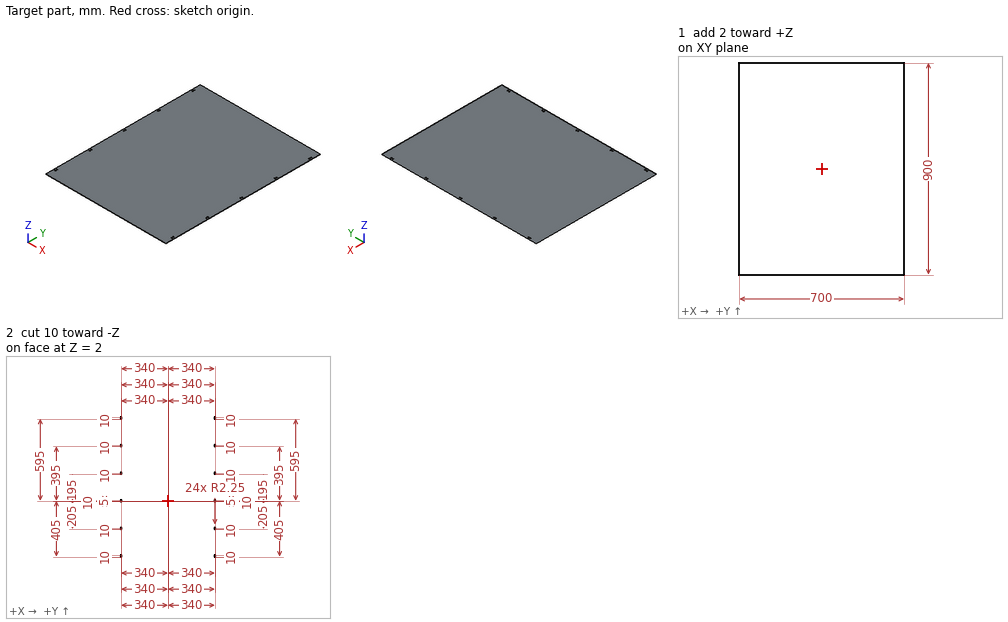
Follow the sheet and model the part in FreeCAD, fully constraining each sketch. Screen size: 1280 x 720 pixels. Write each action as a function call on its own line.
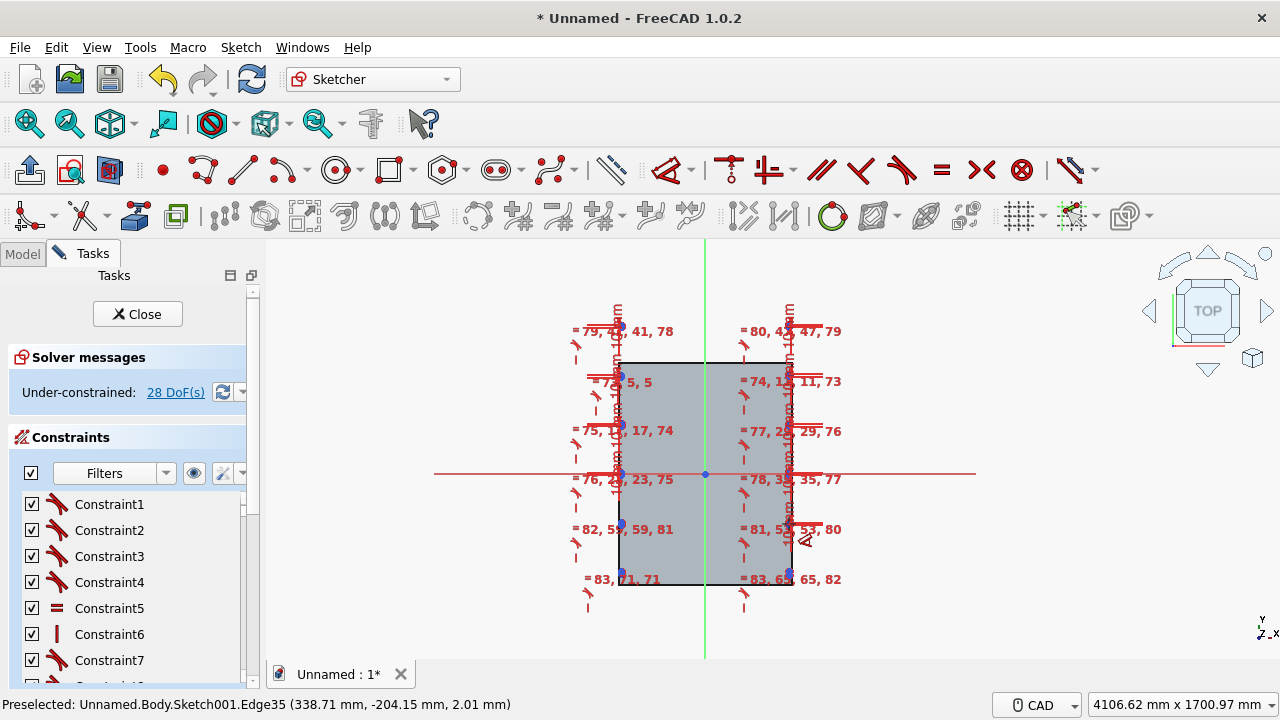
scroll(621, 524, up, 14)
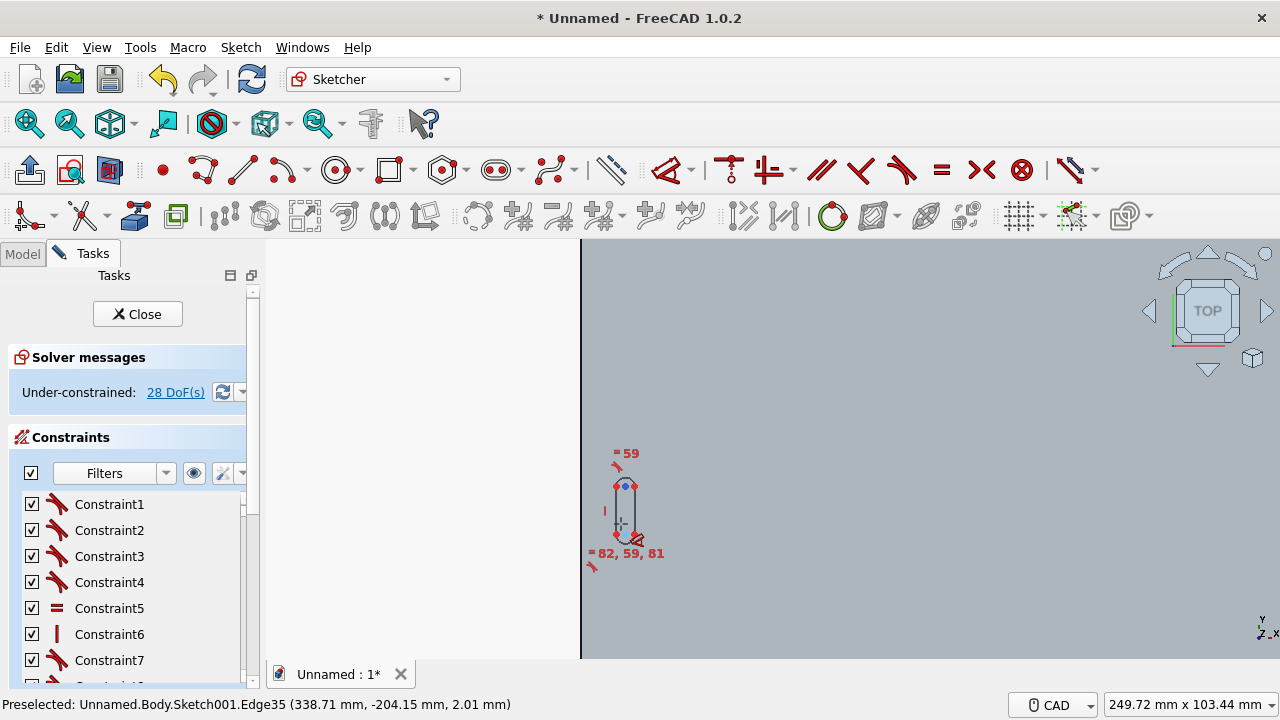
click(616, 520)
click(582, 511)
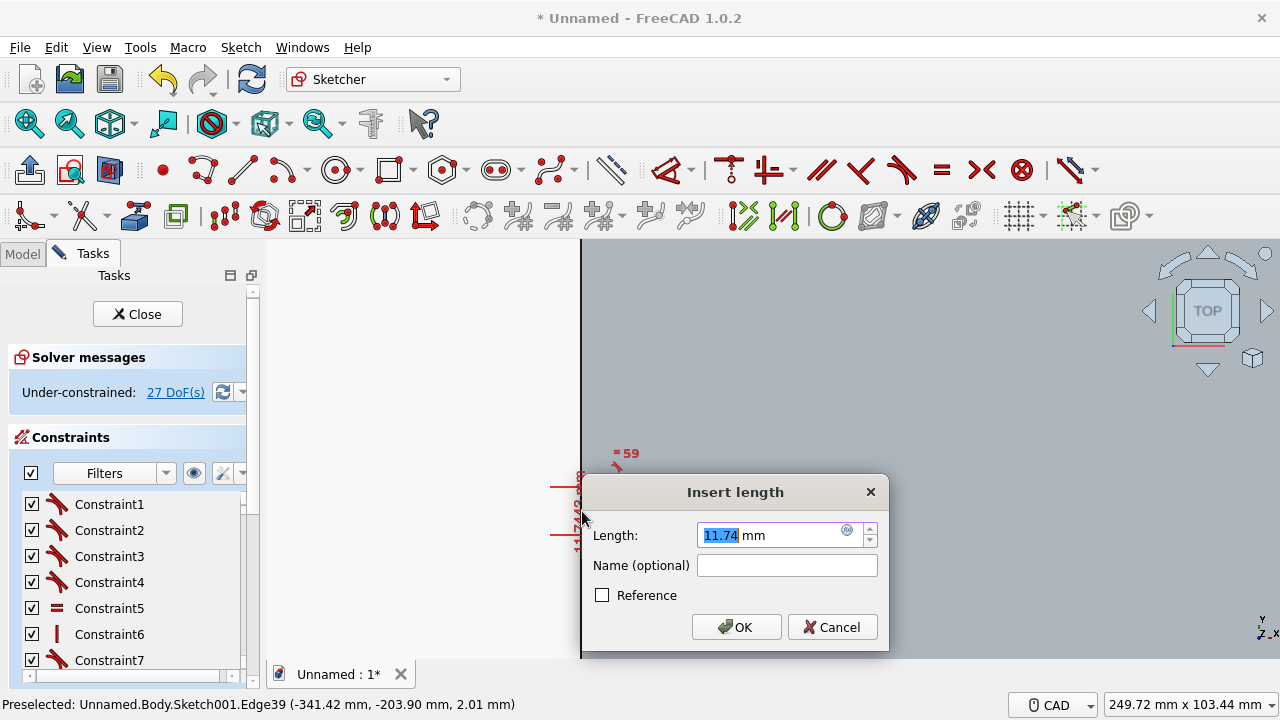
text(10)
key(Return)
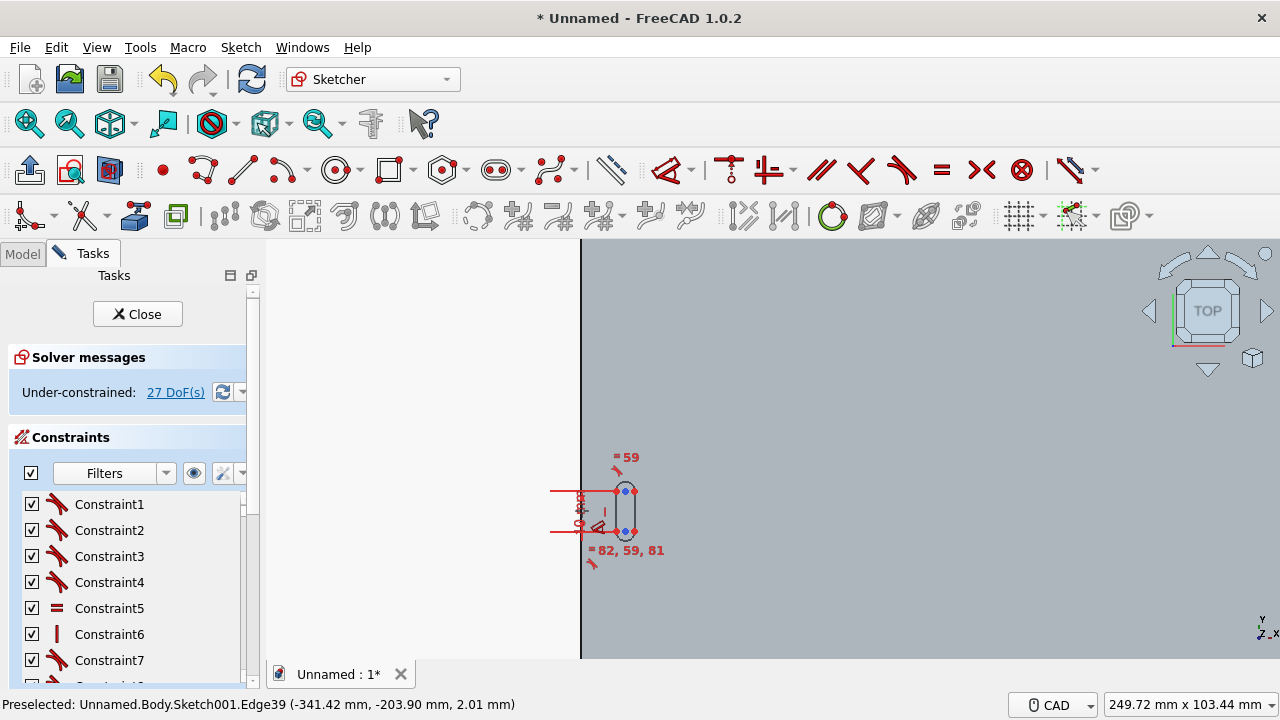
scroll(620, 524, down, 14)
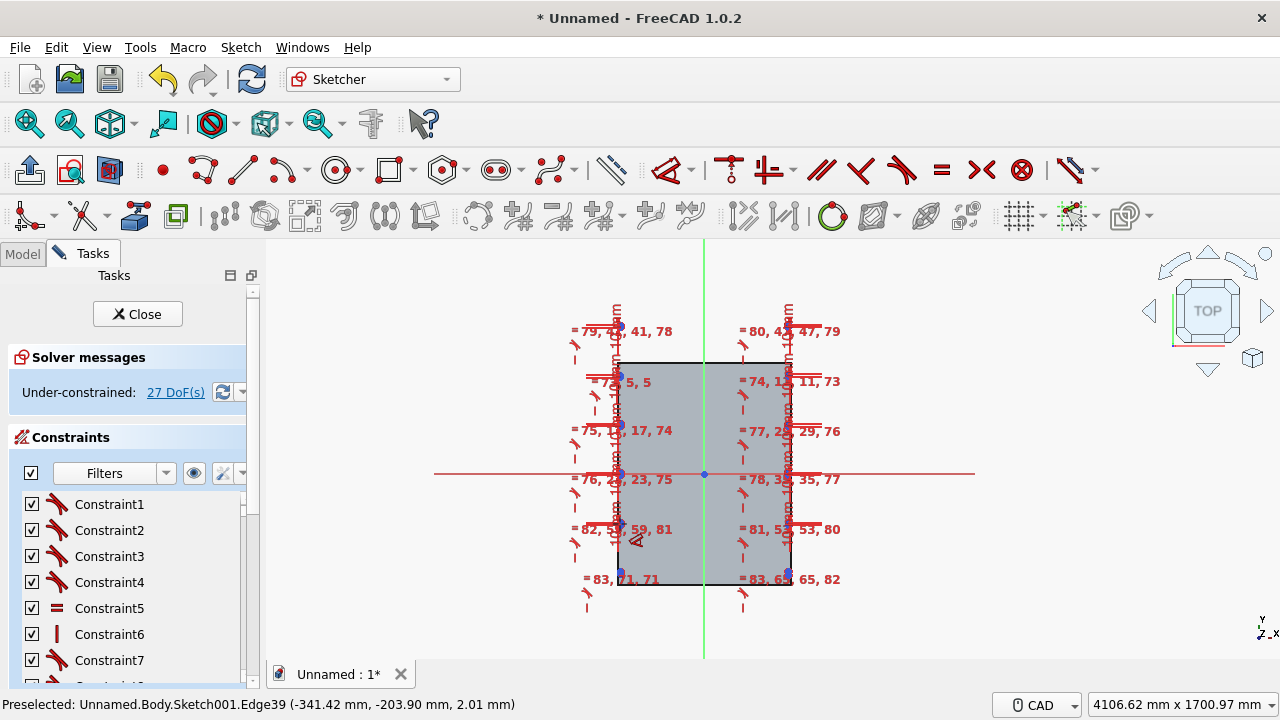
scroll(788, 574, up, 14)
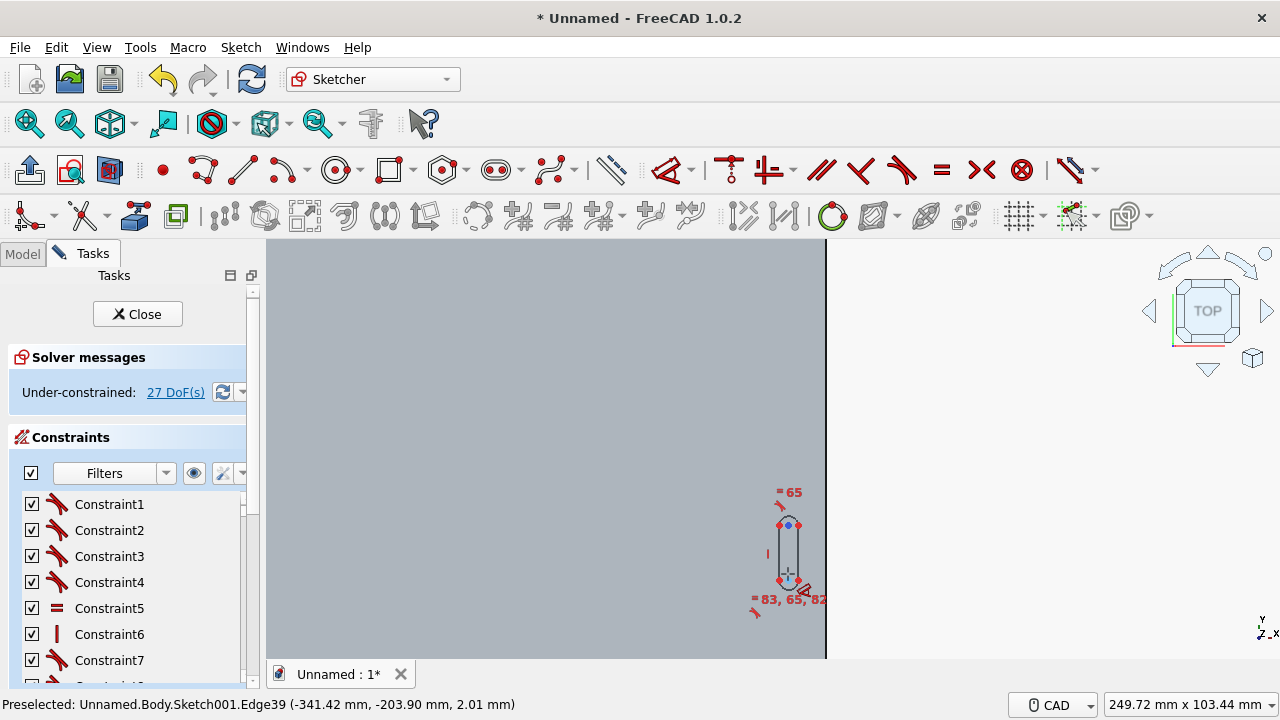
click(779, 564)
click(813, 553)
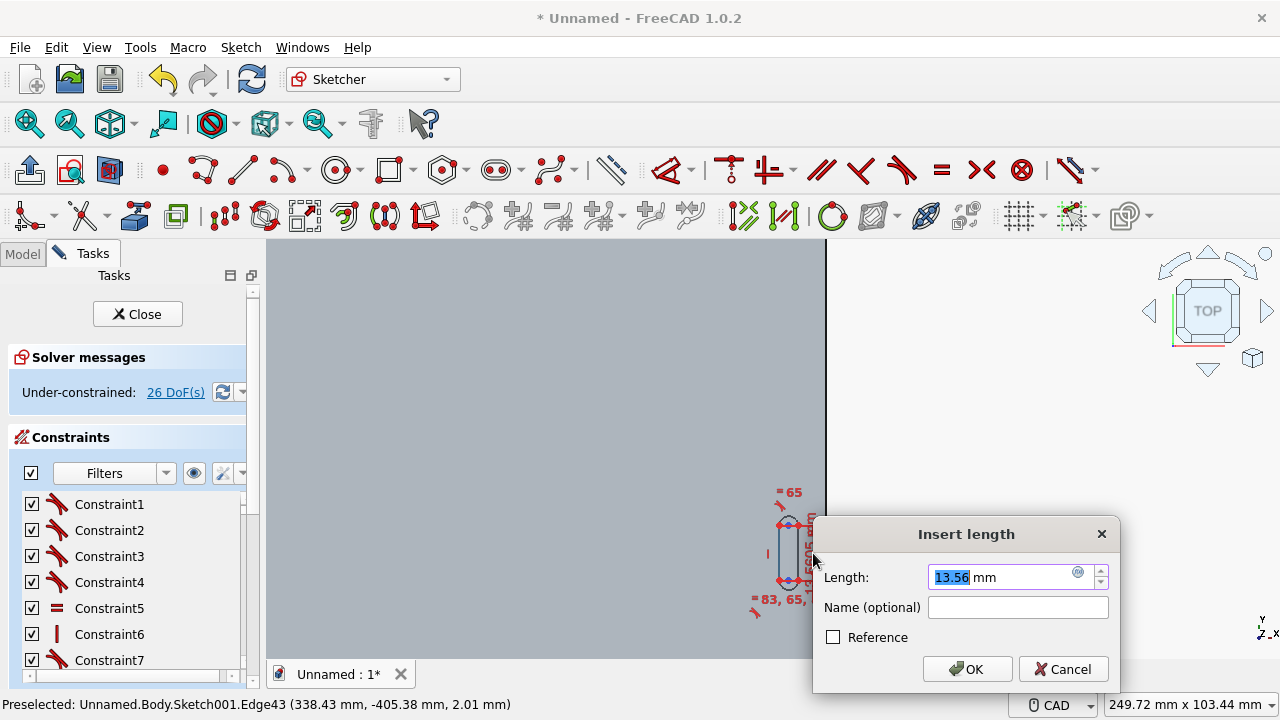
text(10)
key(Return)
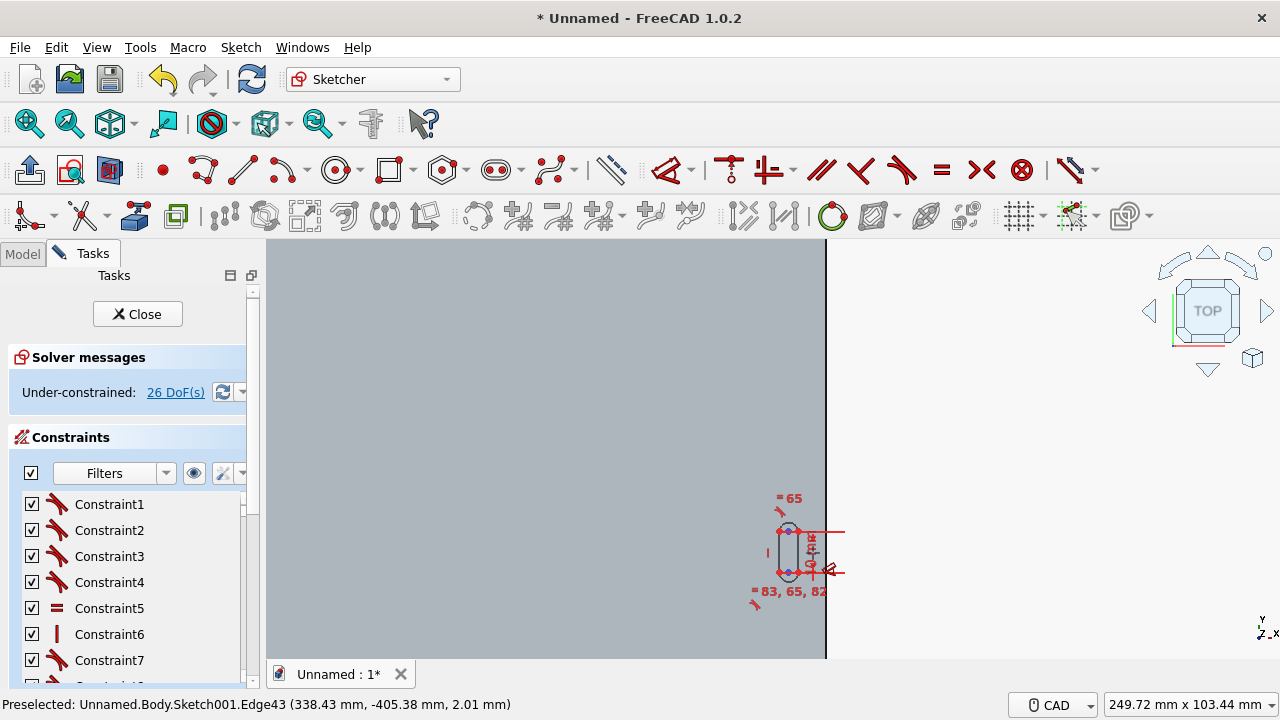
scroll(789, 574, down, 14)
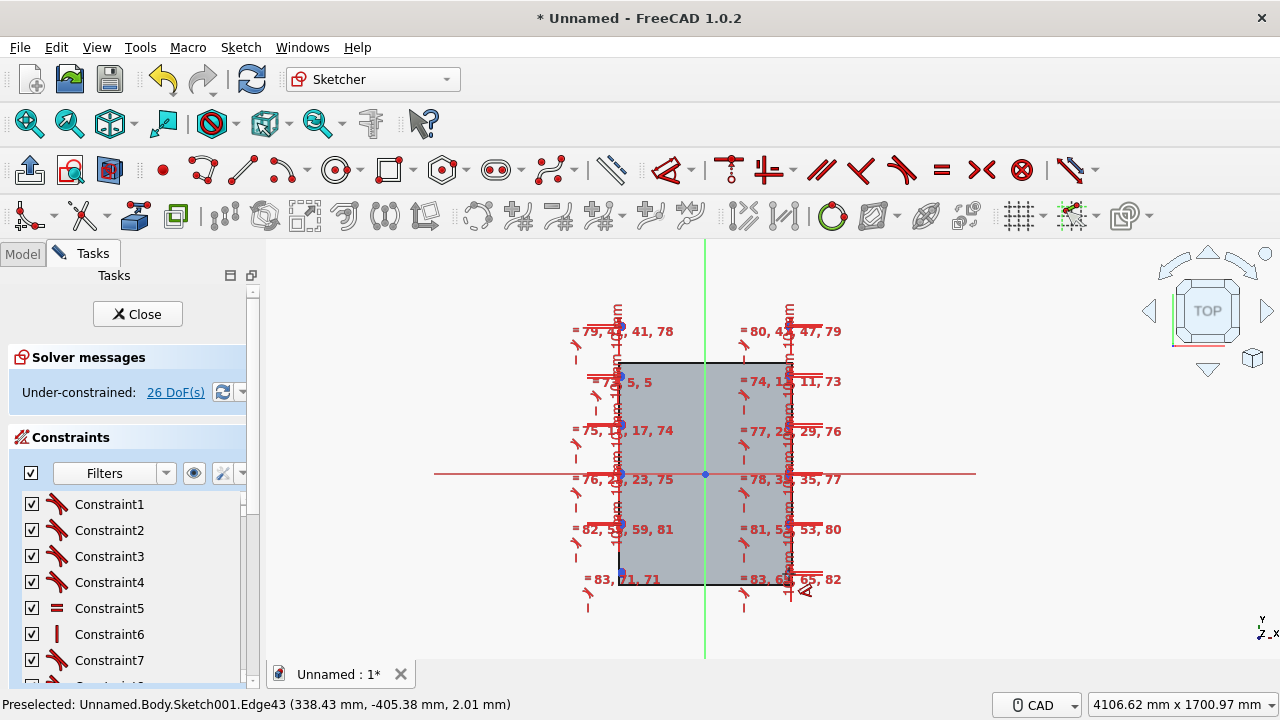
scroll(621, 574, up, 14)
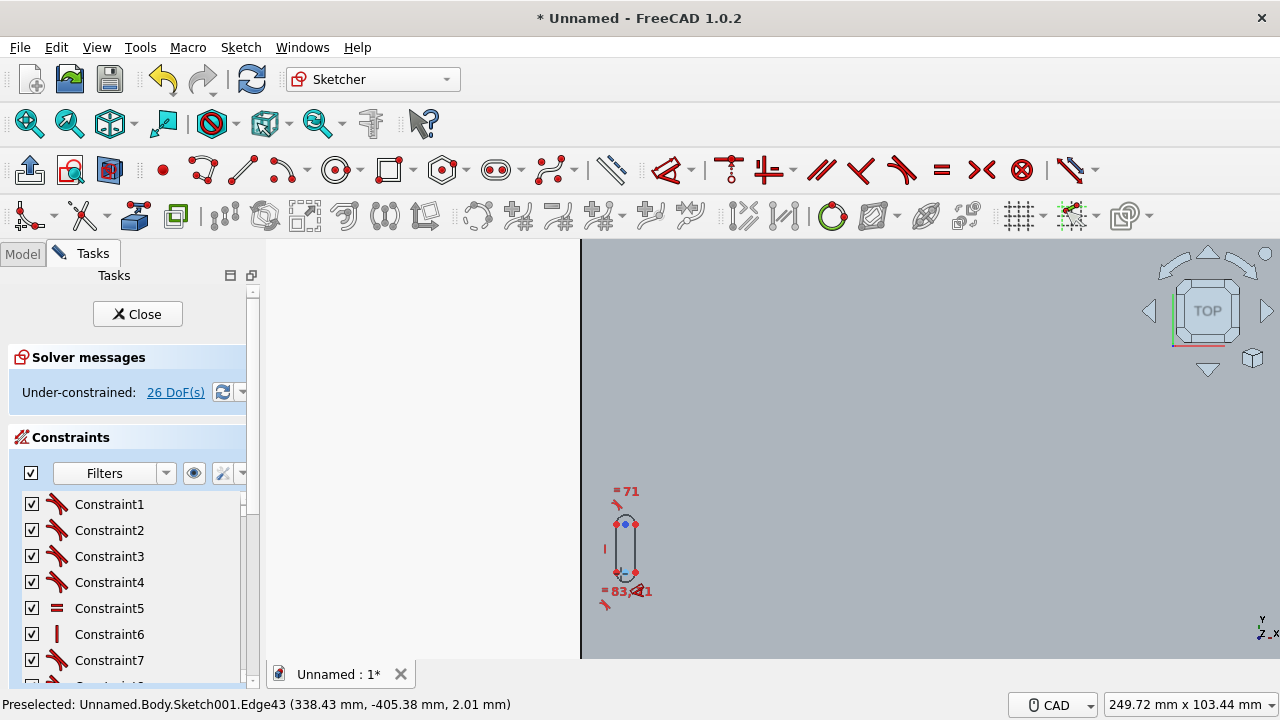
click(616, 558)
click(582, 549)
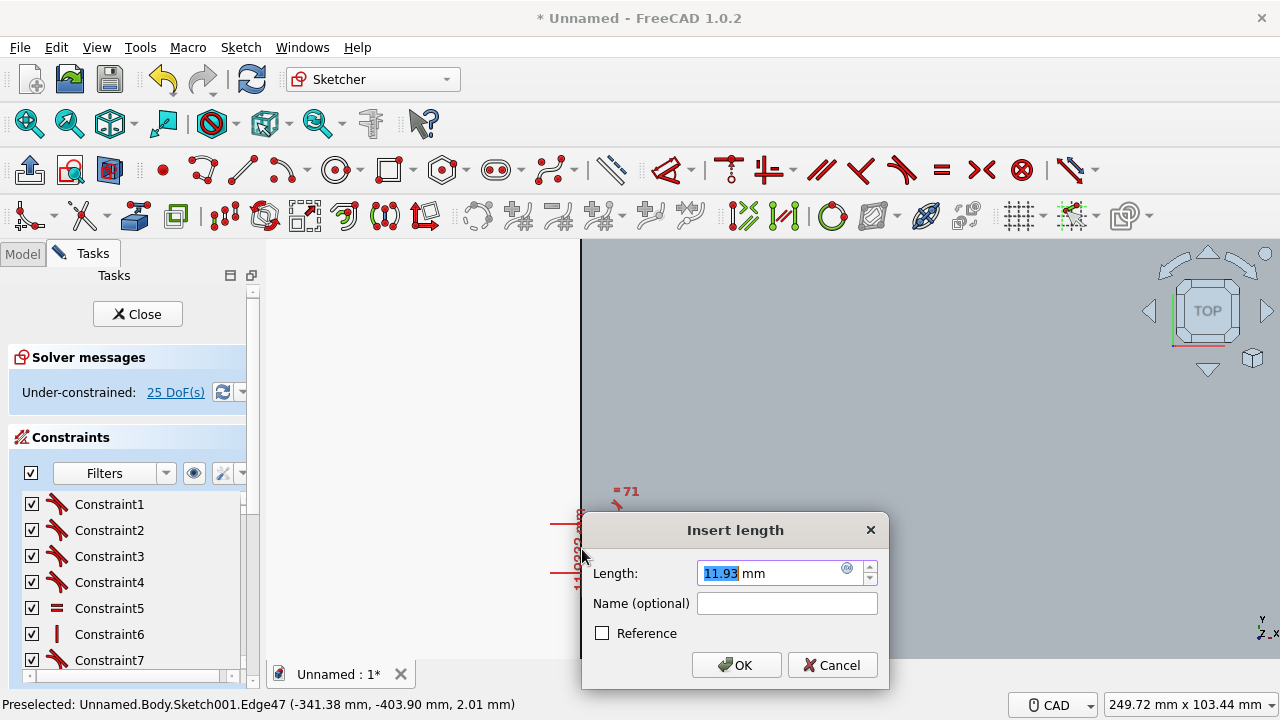
text(10)
key(Return)